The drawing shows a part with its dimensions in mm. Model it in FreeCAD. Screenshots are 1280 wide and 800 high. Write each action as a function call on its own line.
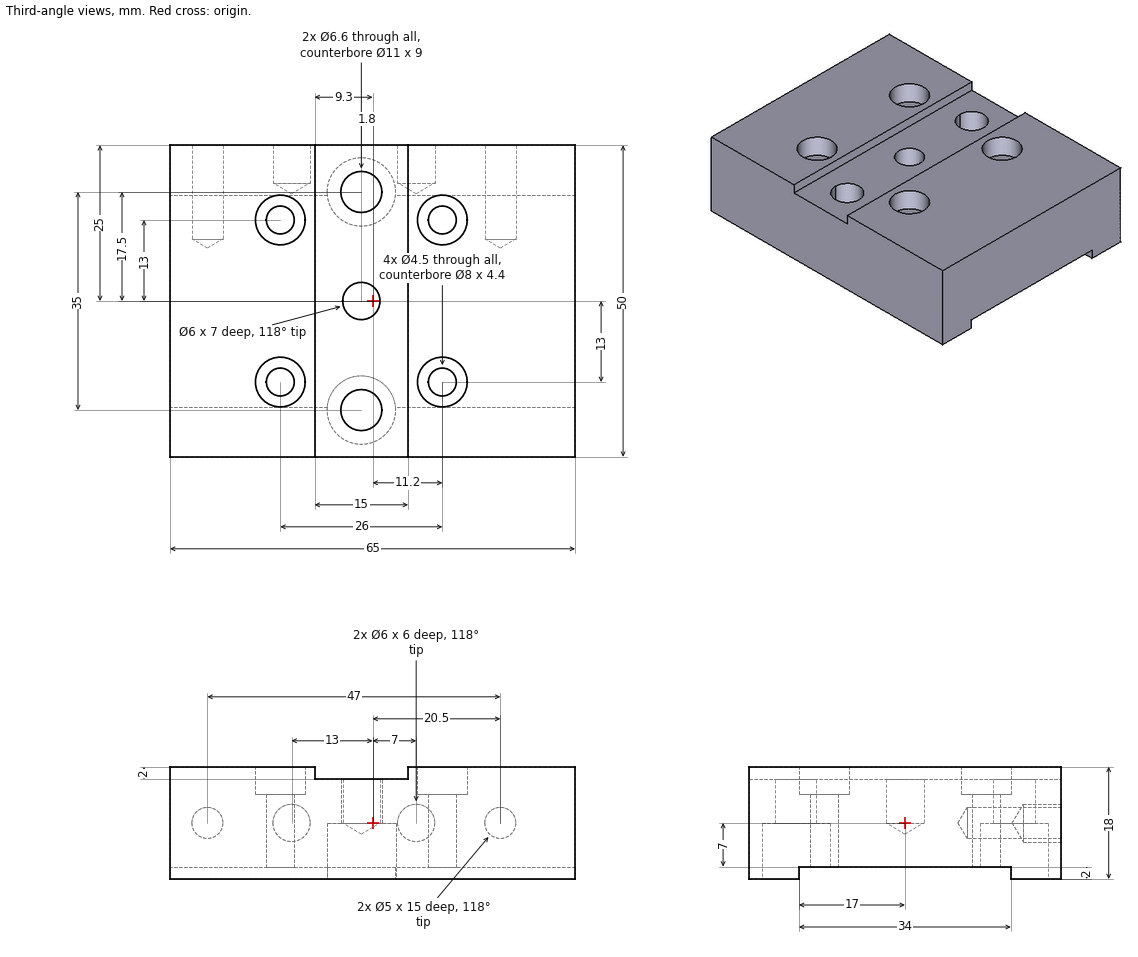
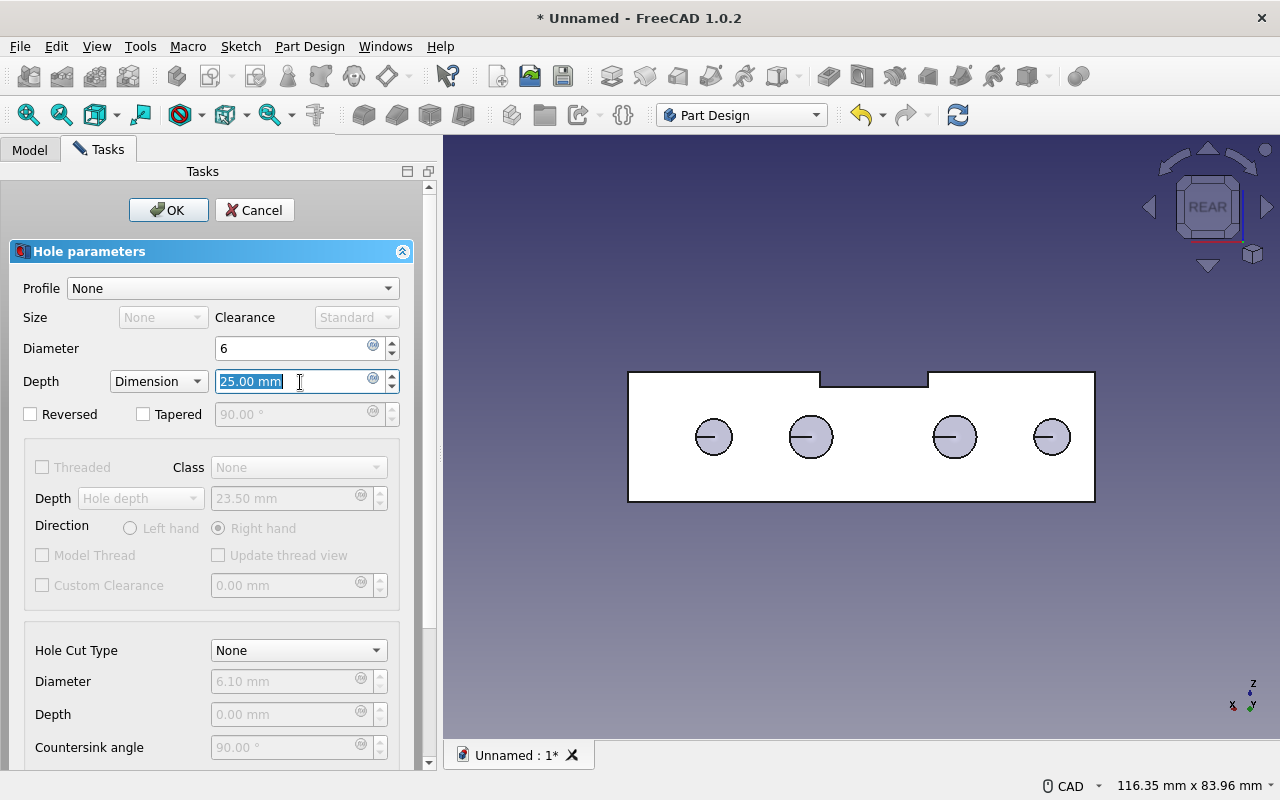
text(6)
key(Tab)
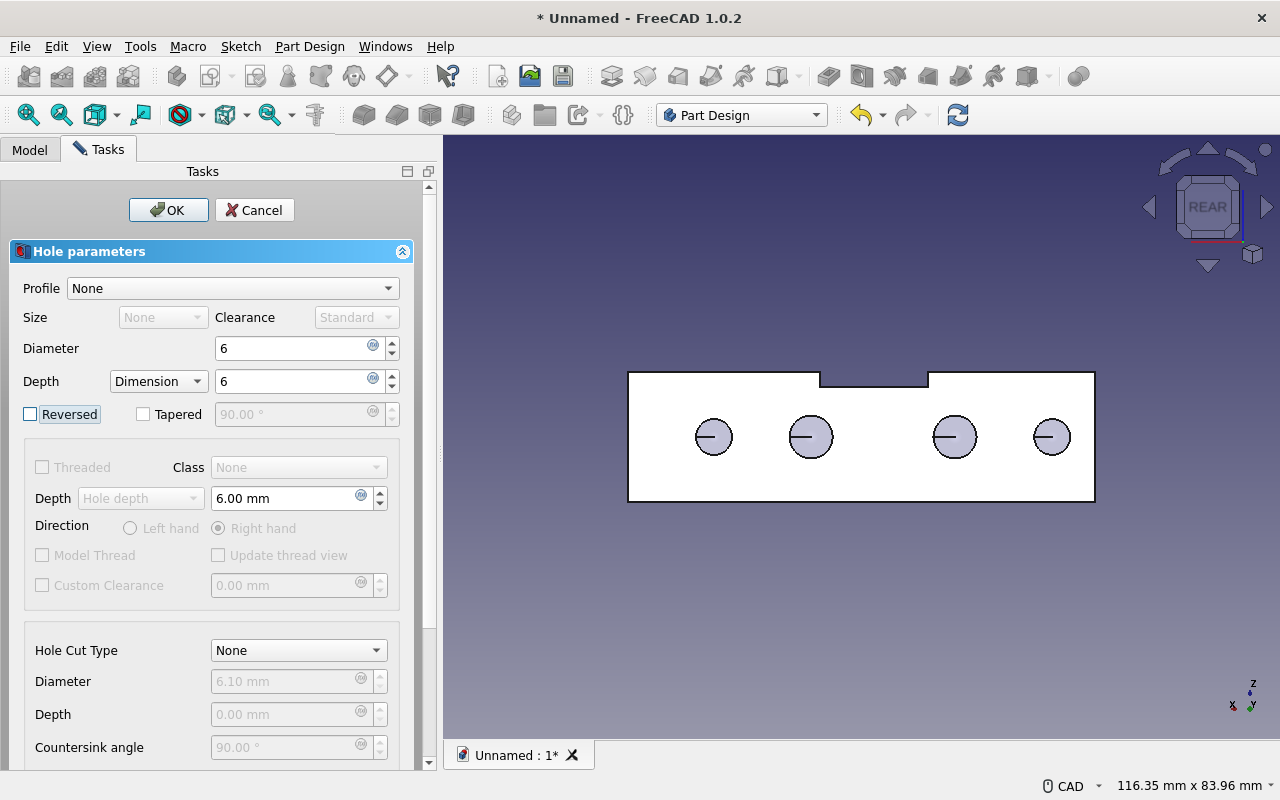
click(169, 210)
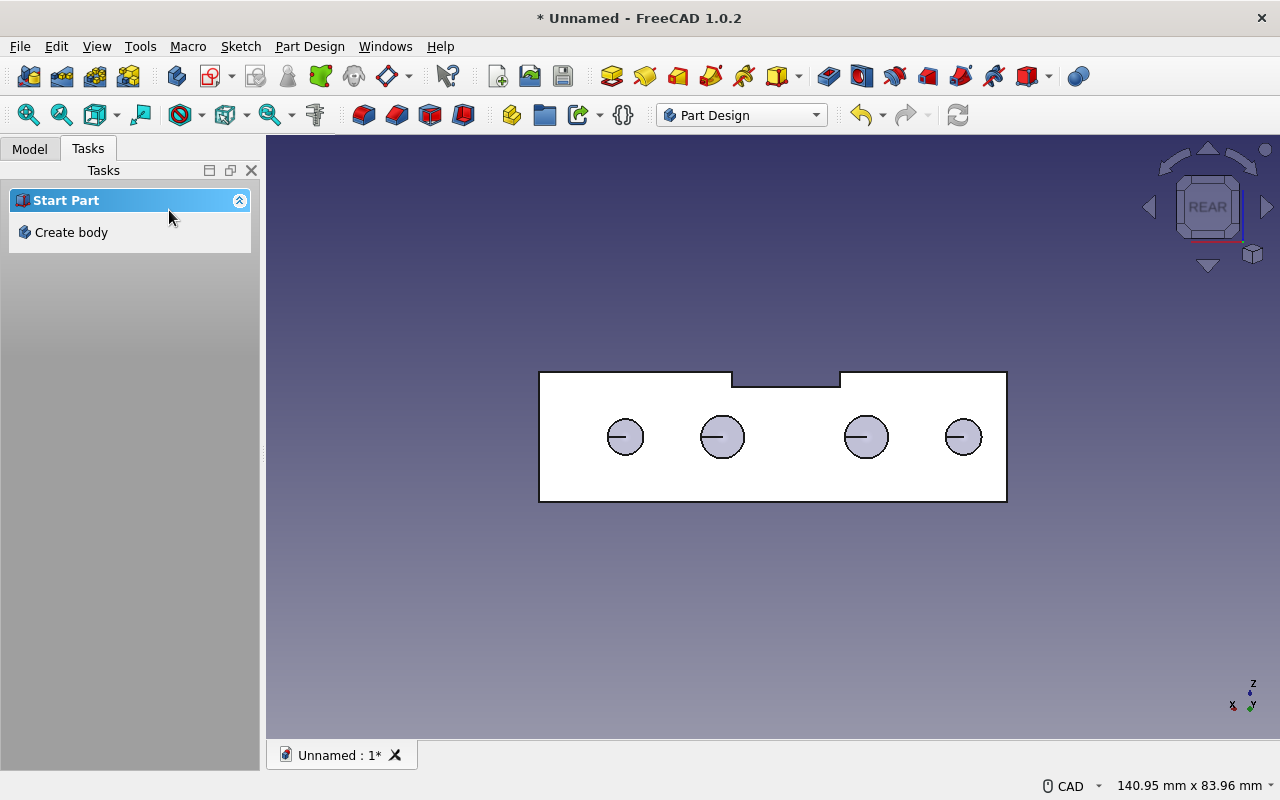
key(0)